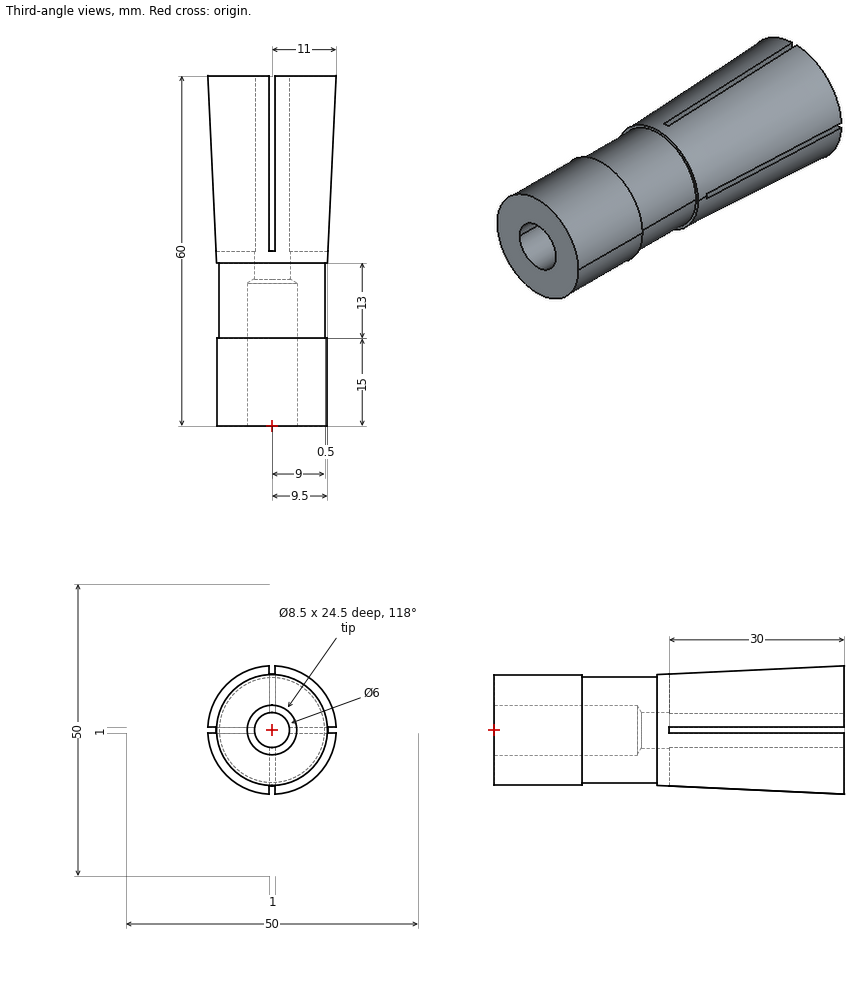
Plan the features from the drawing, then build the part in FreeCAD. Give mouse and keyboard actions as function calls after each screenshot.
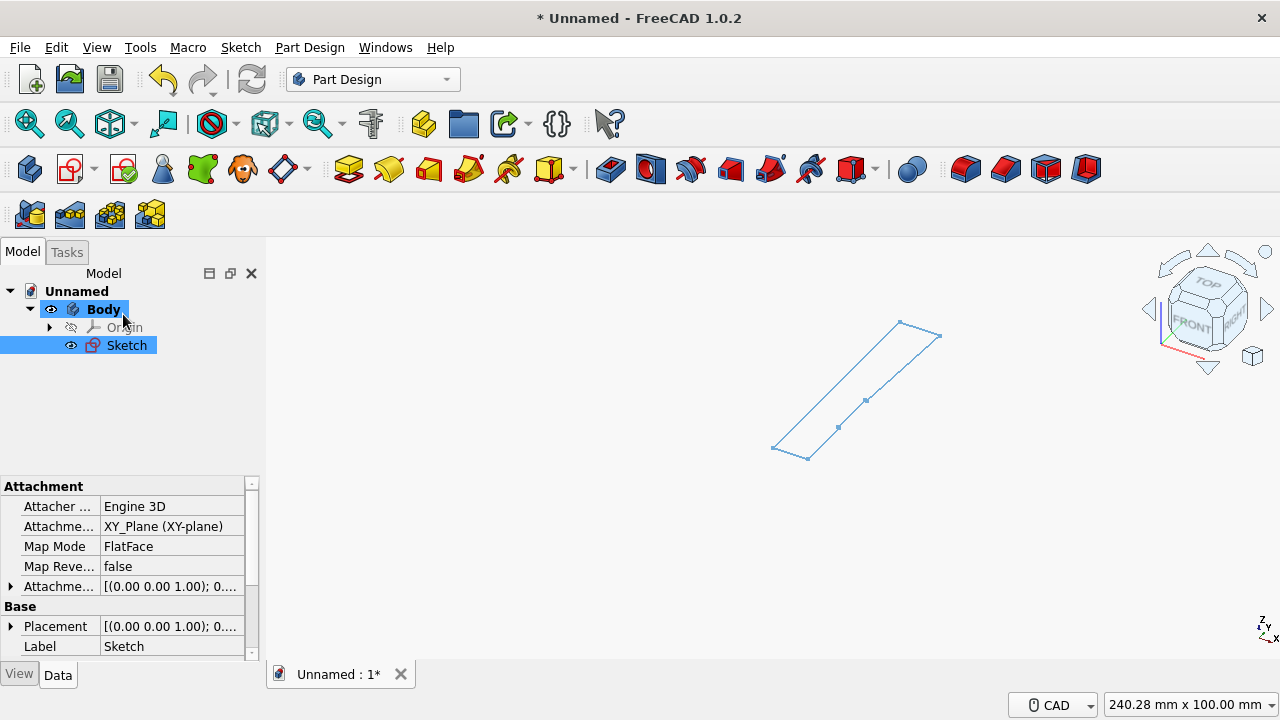
click(390, 170)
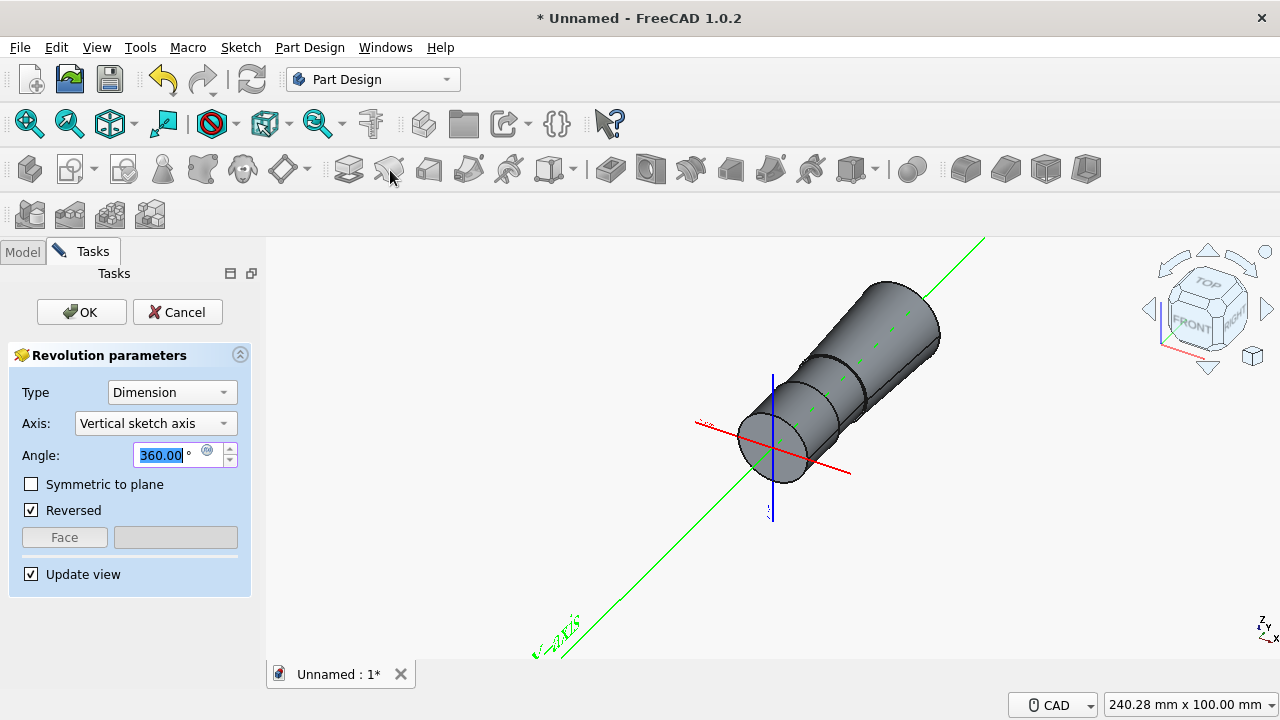
click(82, 312)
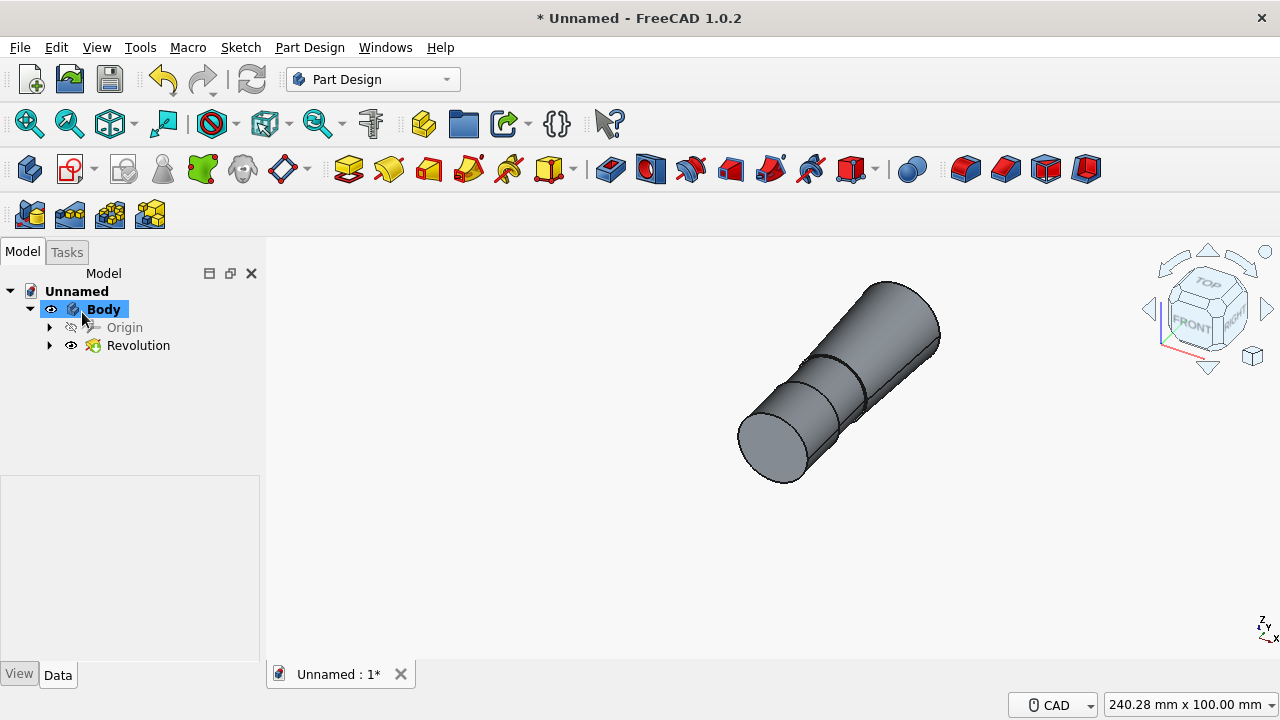
key(4)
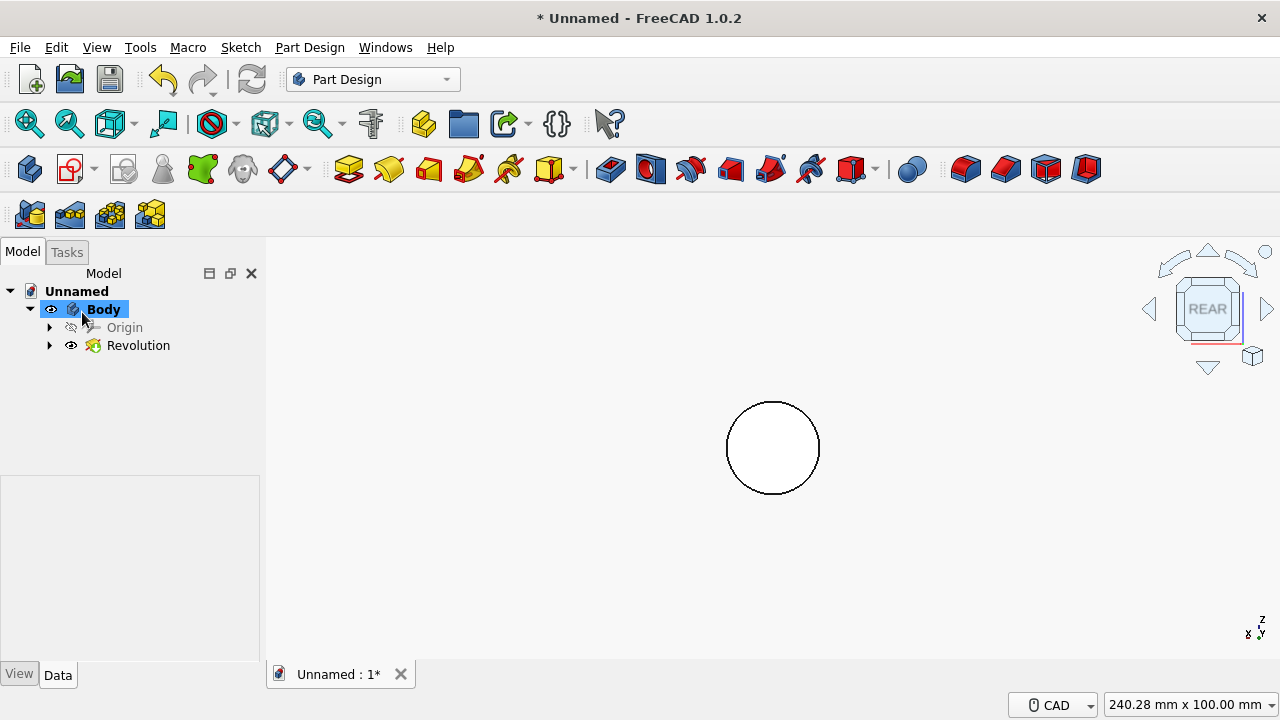
key(v)
key(f)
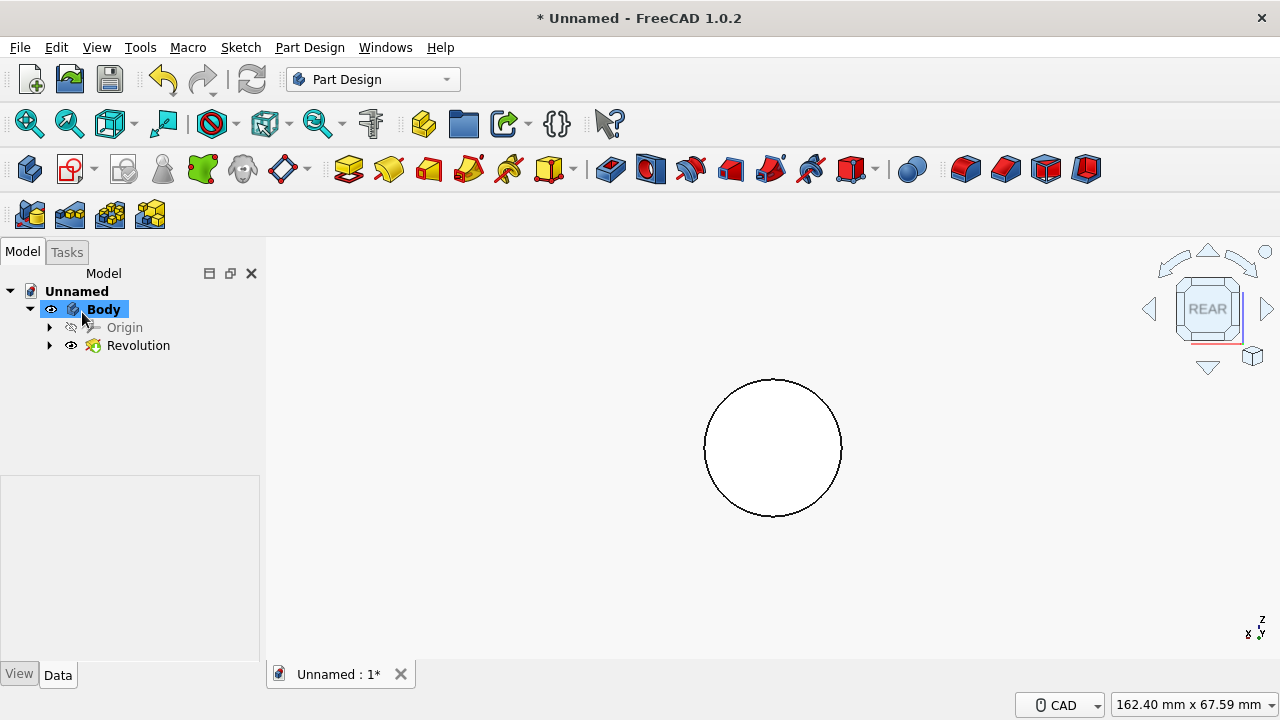
click(773, 447)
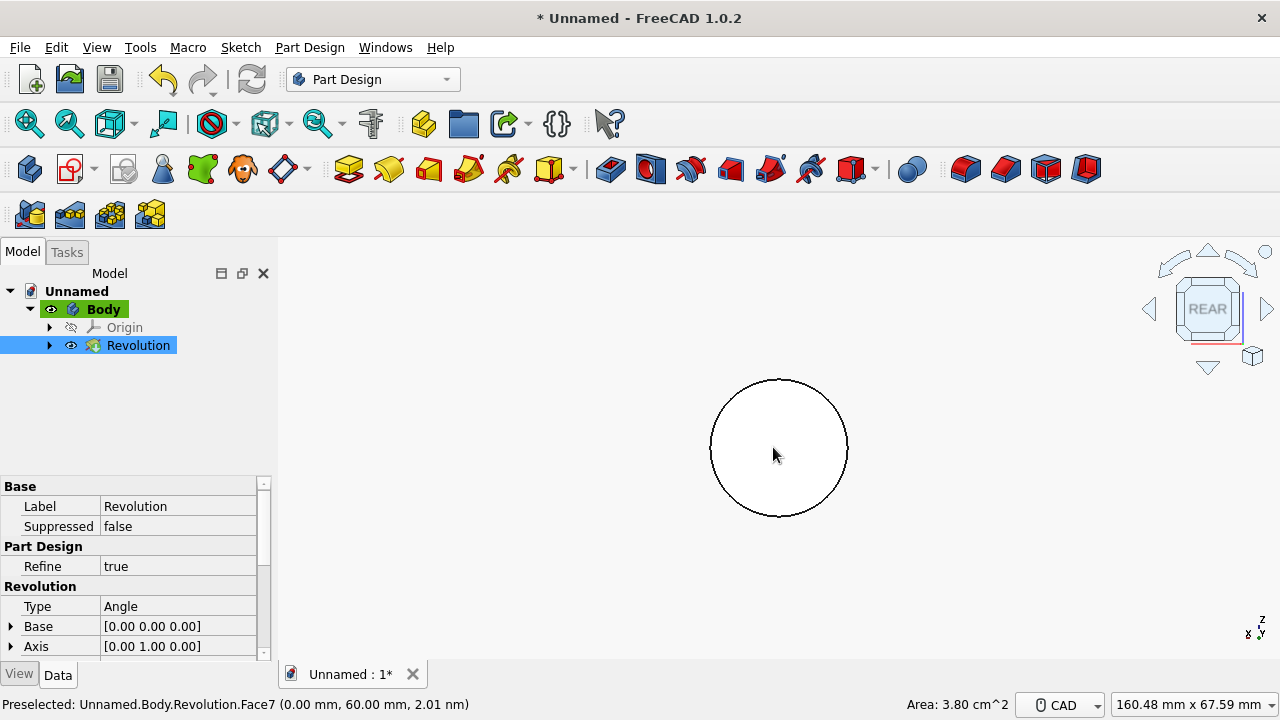
click(70, 170)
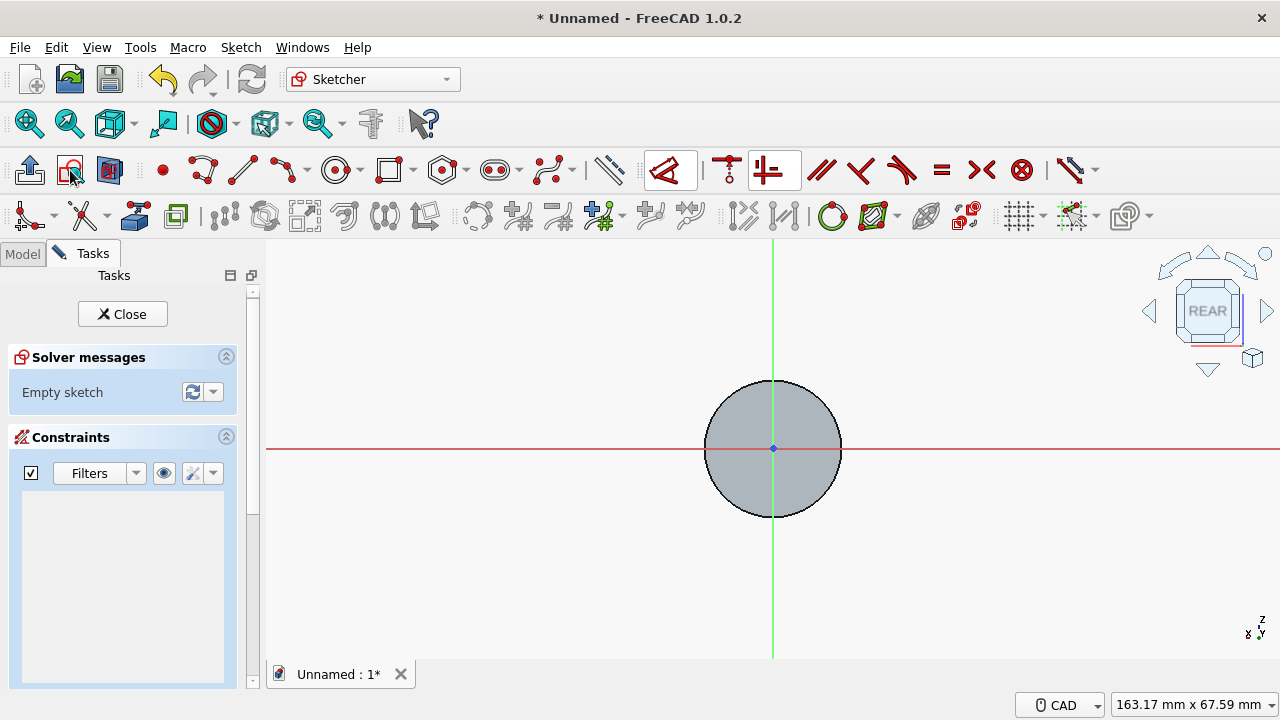
scroll(784, 449, up, 10)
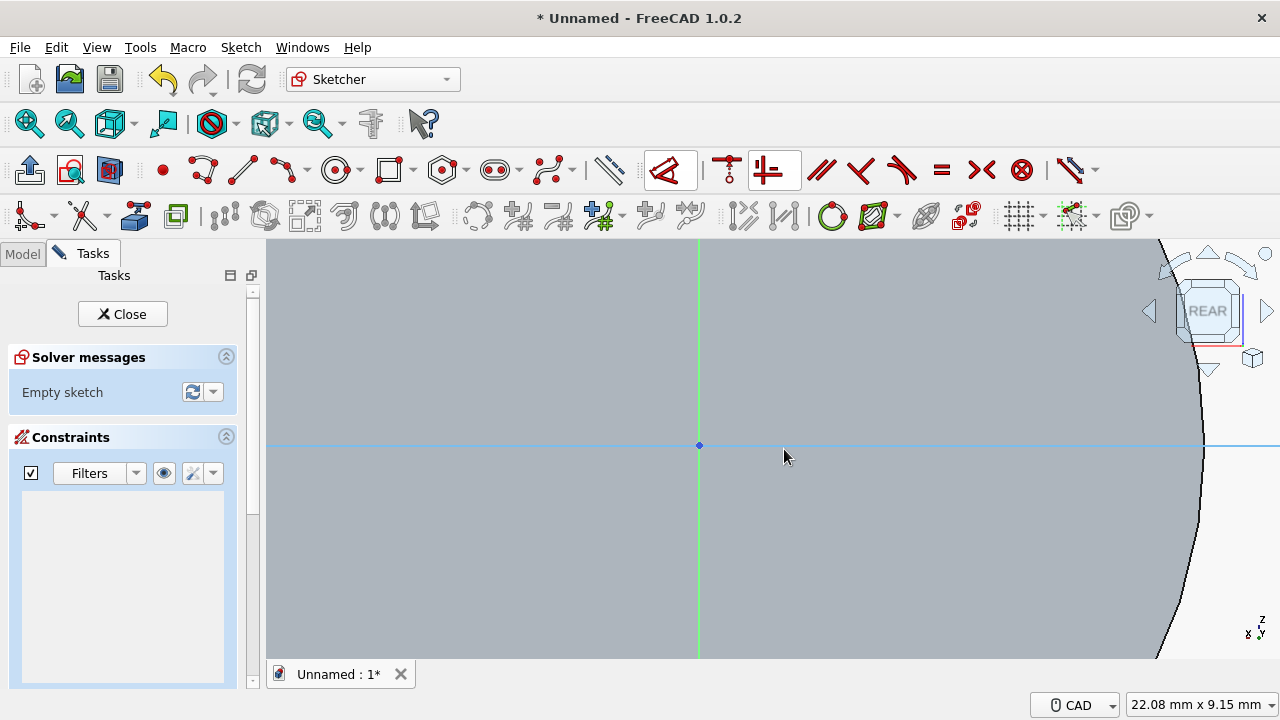
key(g)
key(c)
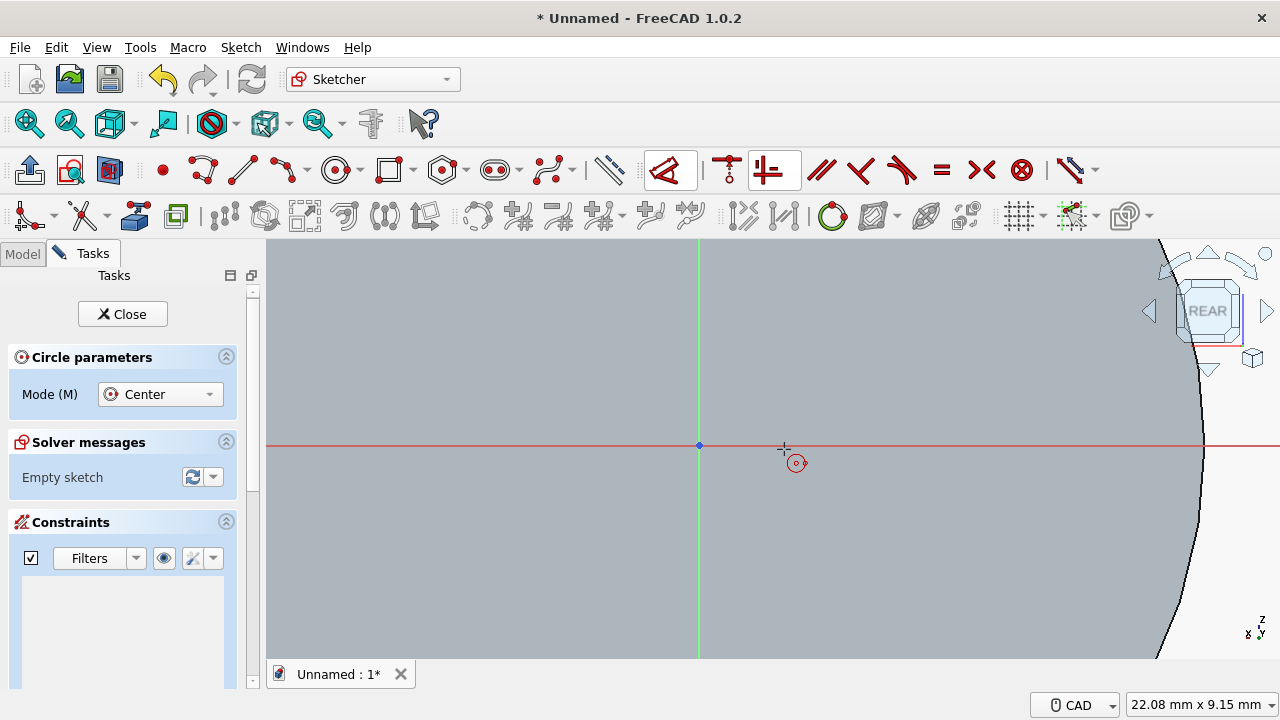
click(699, 446)
move(797, 348)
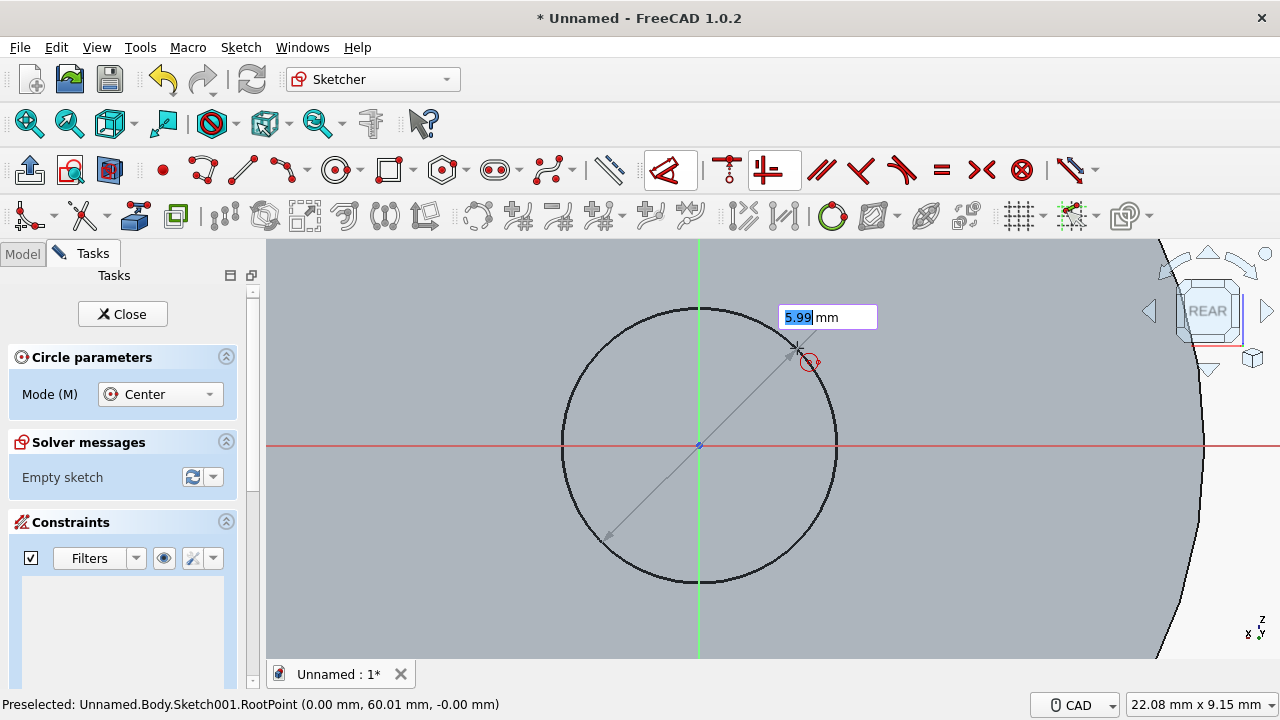
text(6)
key(Return)
key(Escape)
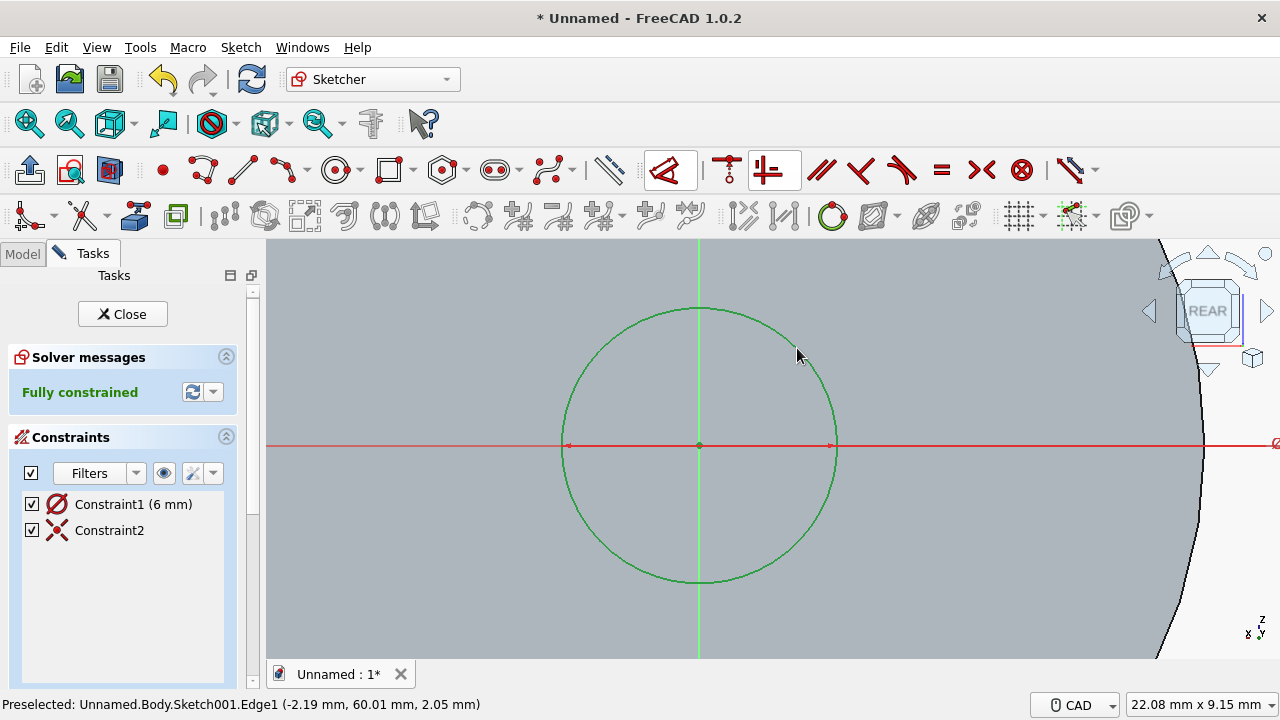
click(123, 314)